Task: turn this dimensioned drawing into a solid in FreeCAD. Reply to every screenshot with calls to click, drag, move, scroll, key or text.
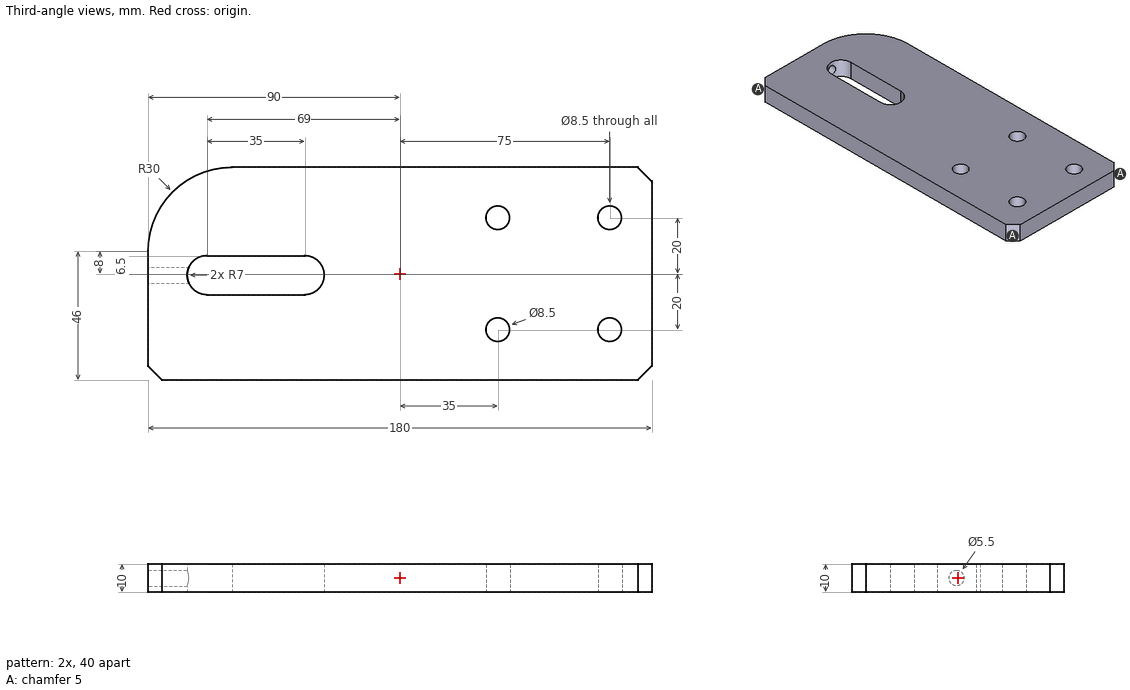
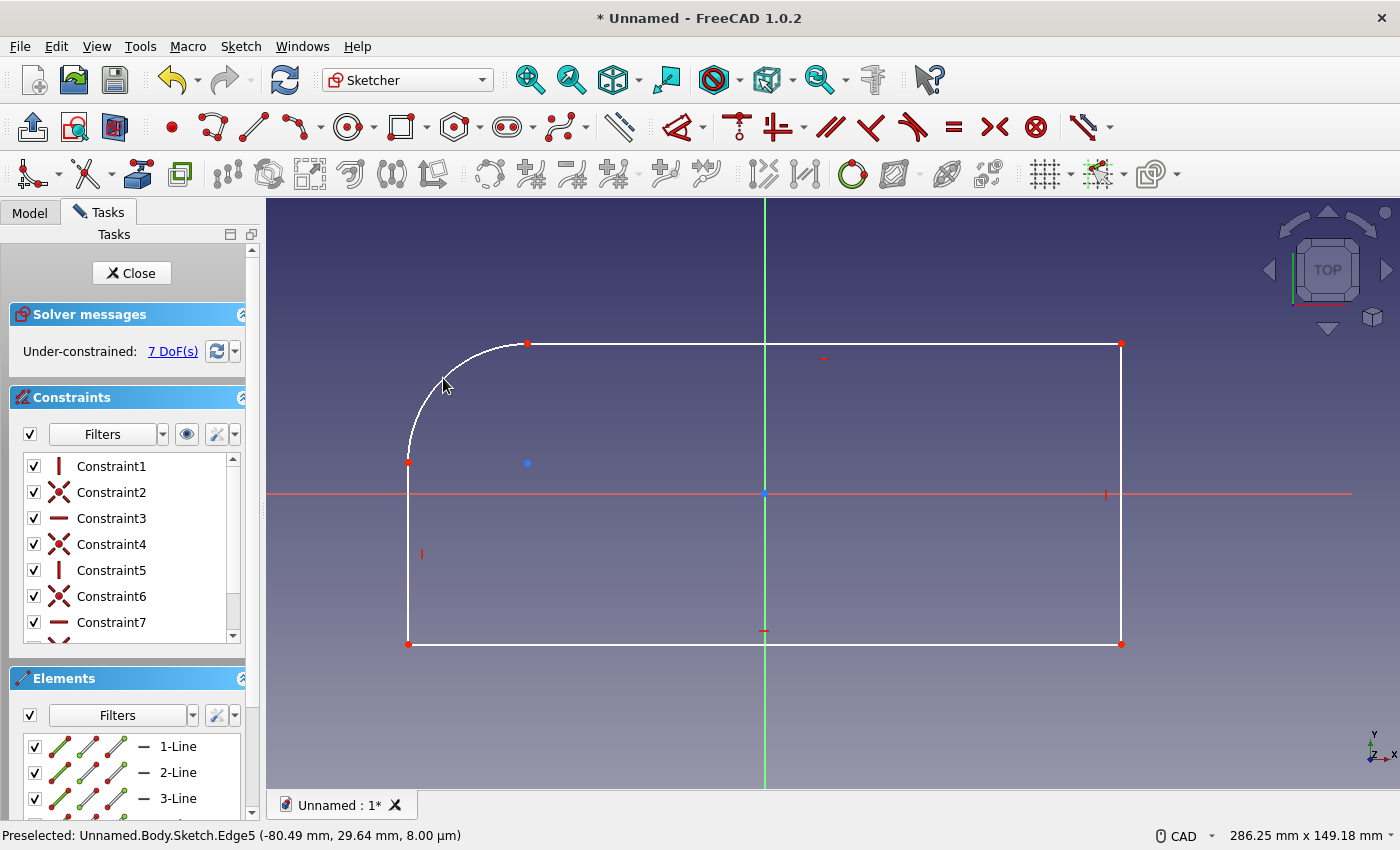
click(408, 518)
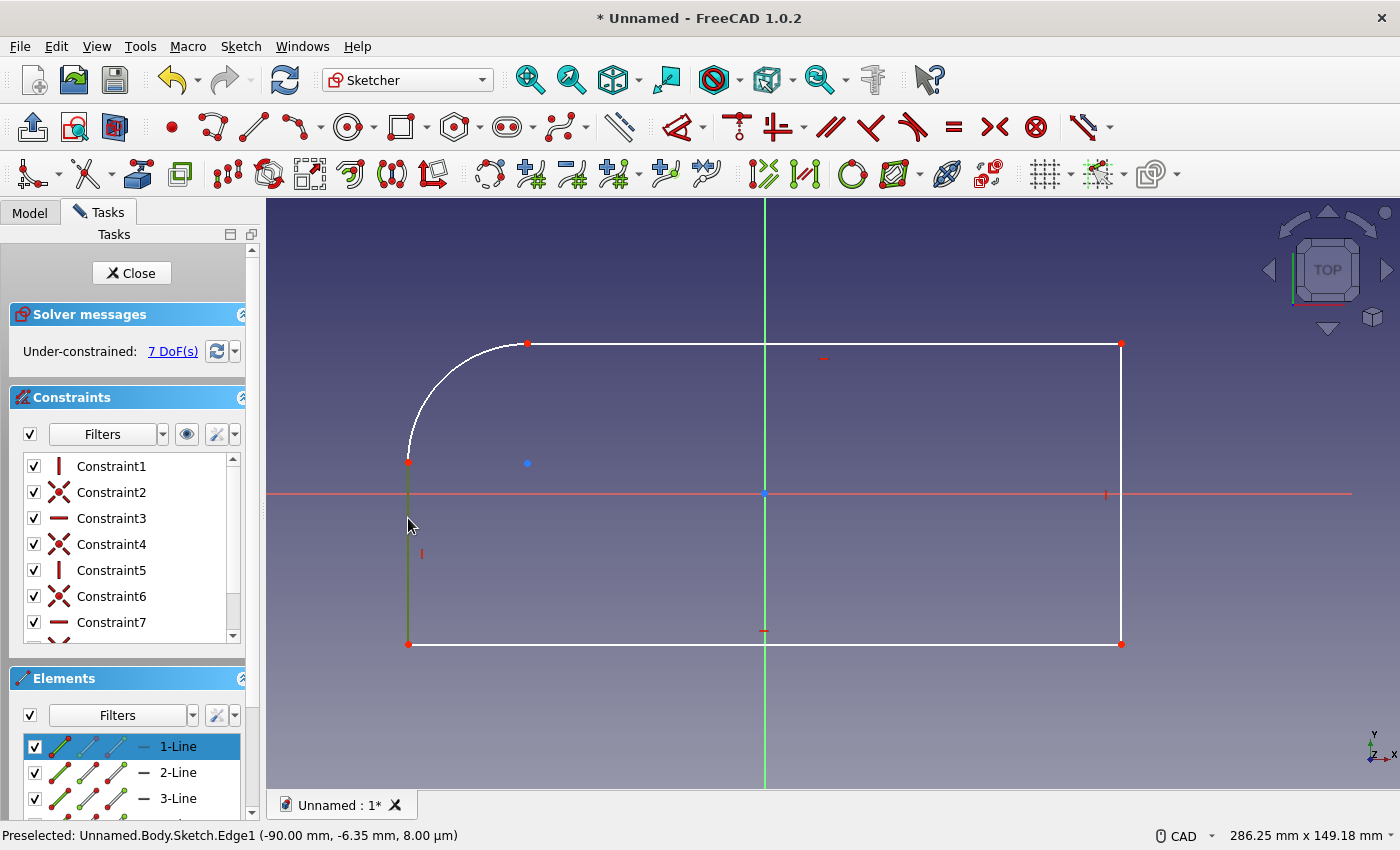
click(473, 357)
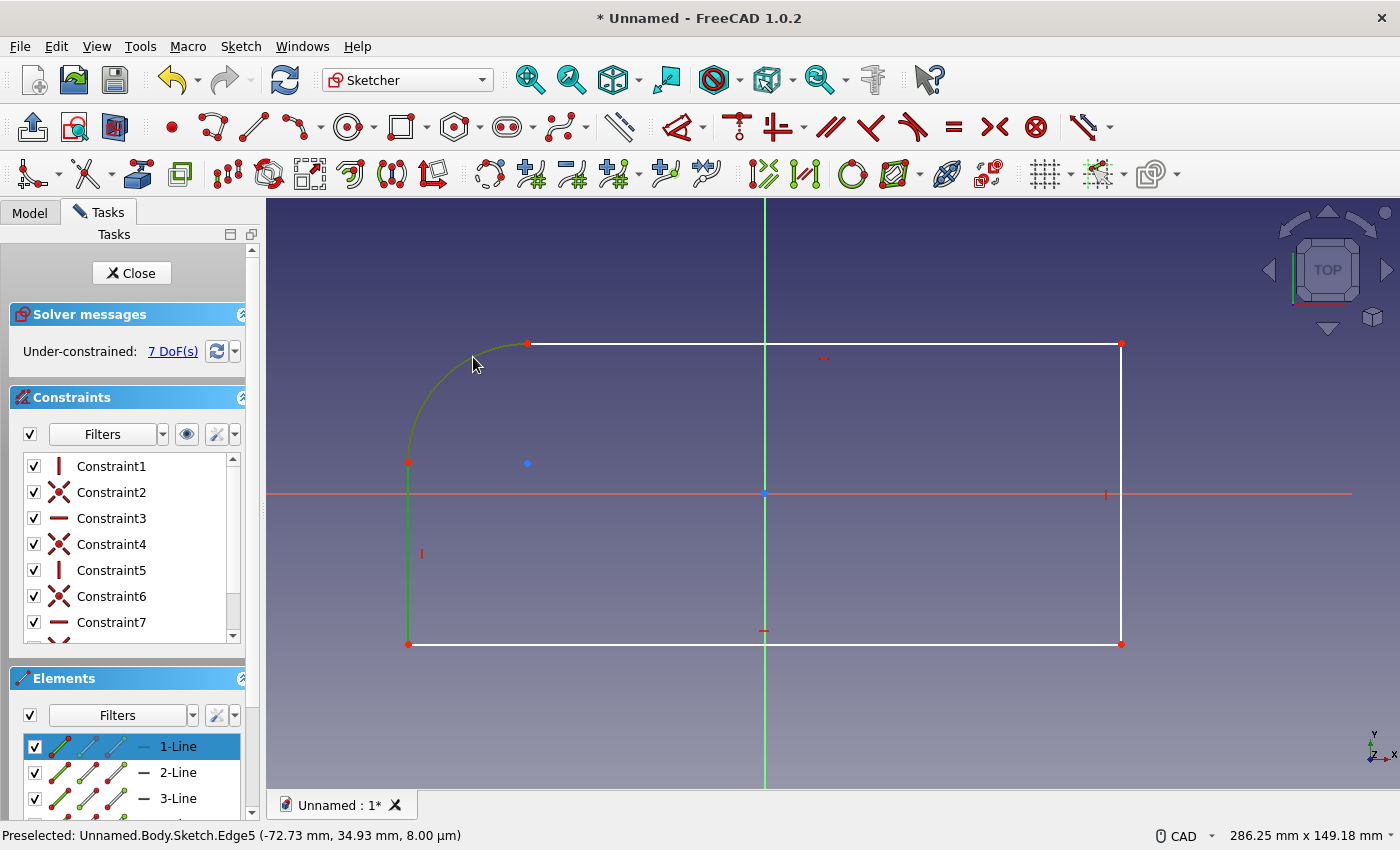
click(913, 128)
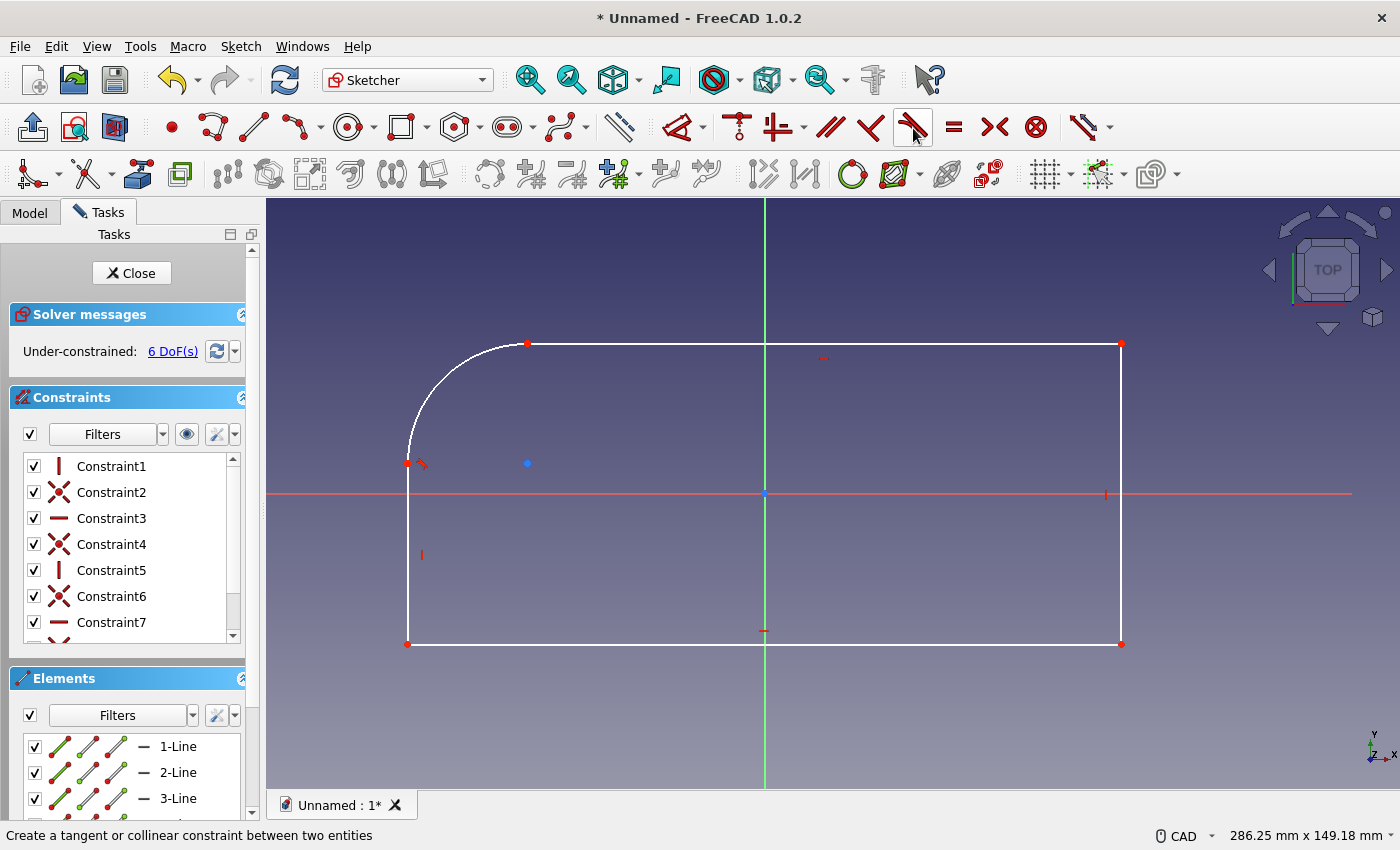
click(943, 344)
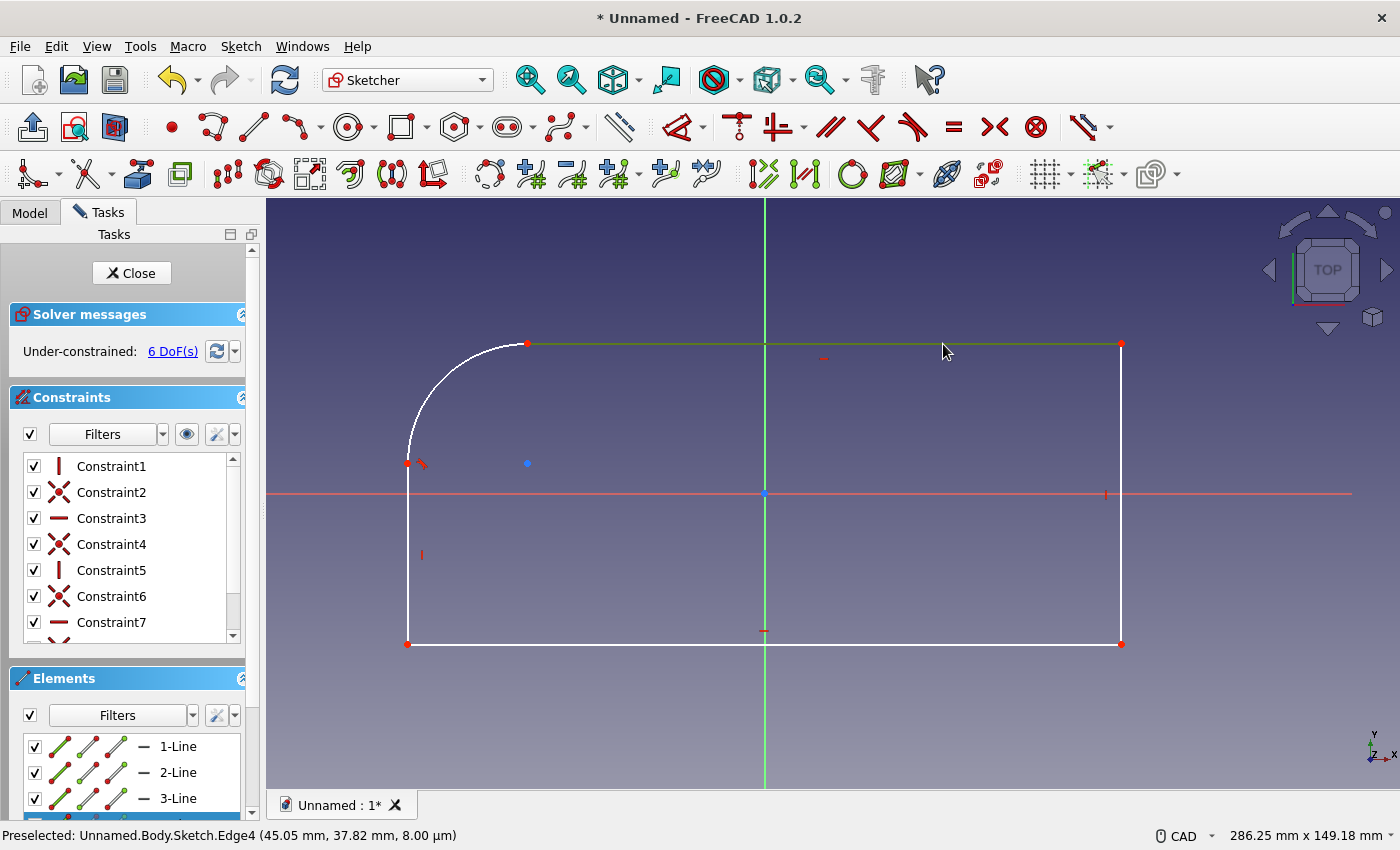
click(473, 357)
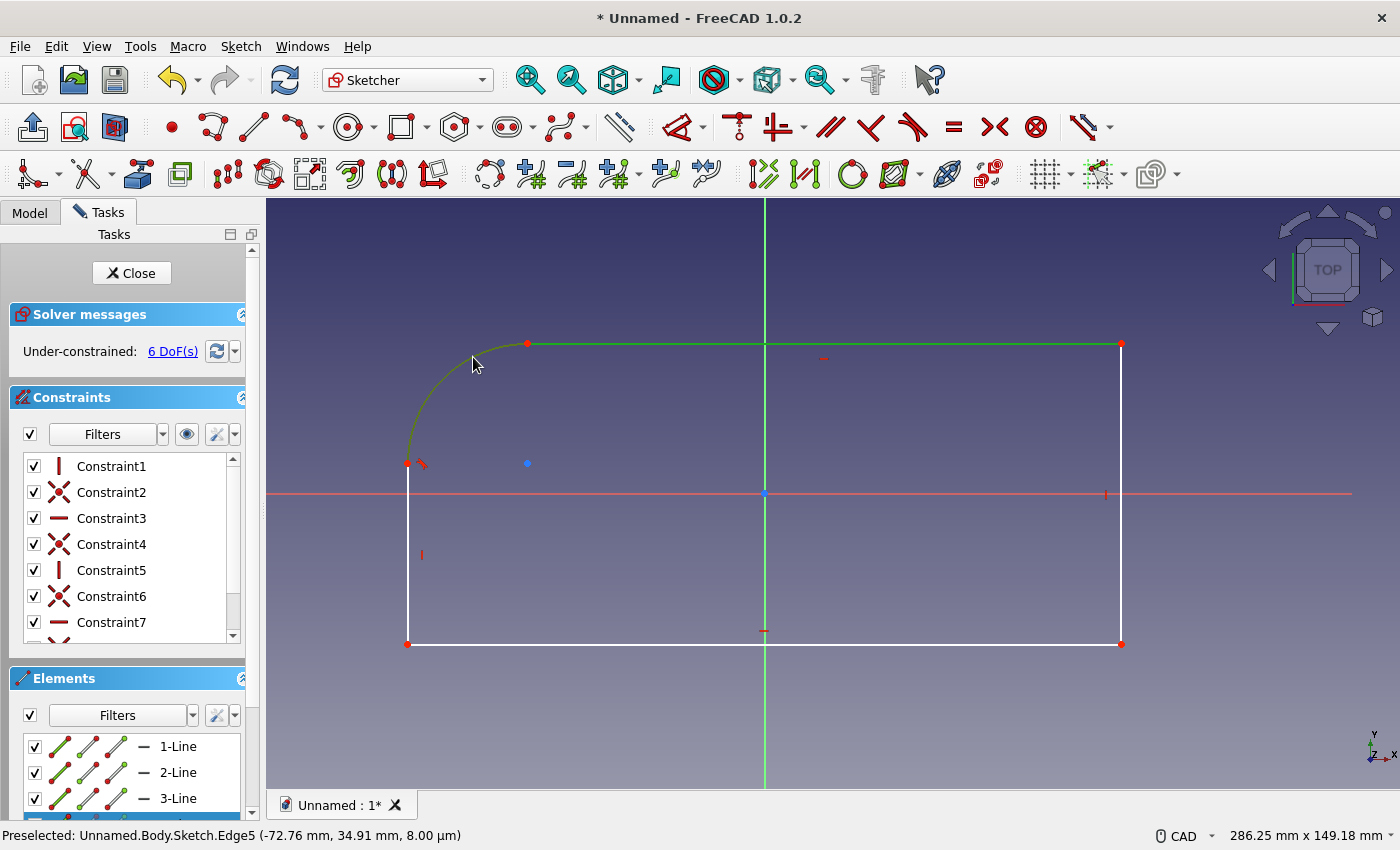
click(913, 128)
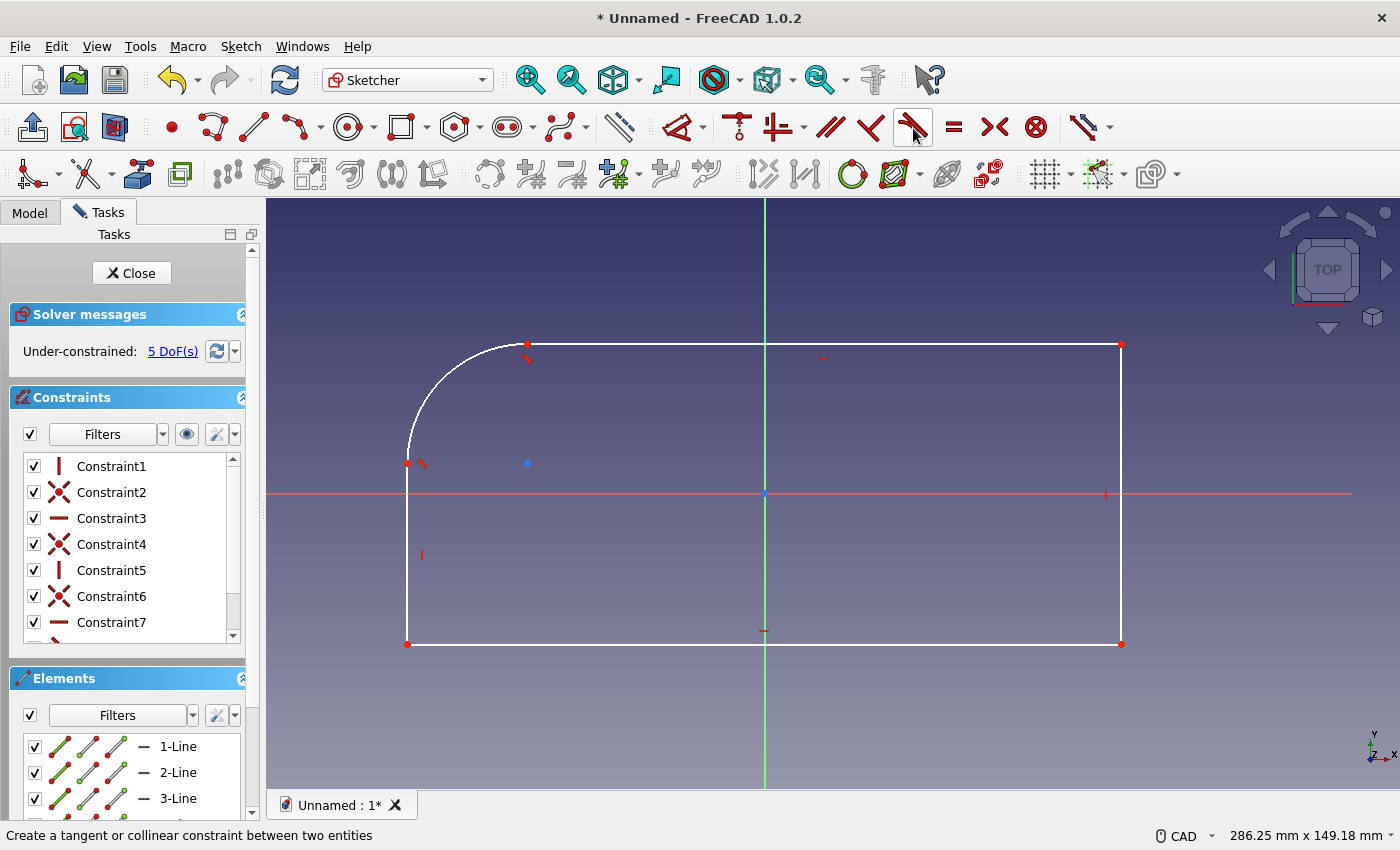
click(473, 357)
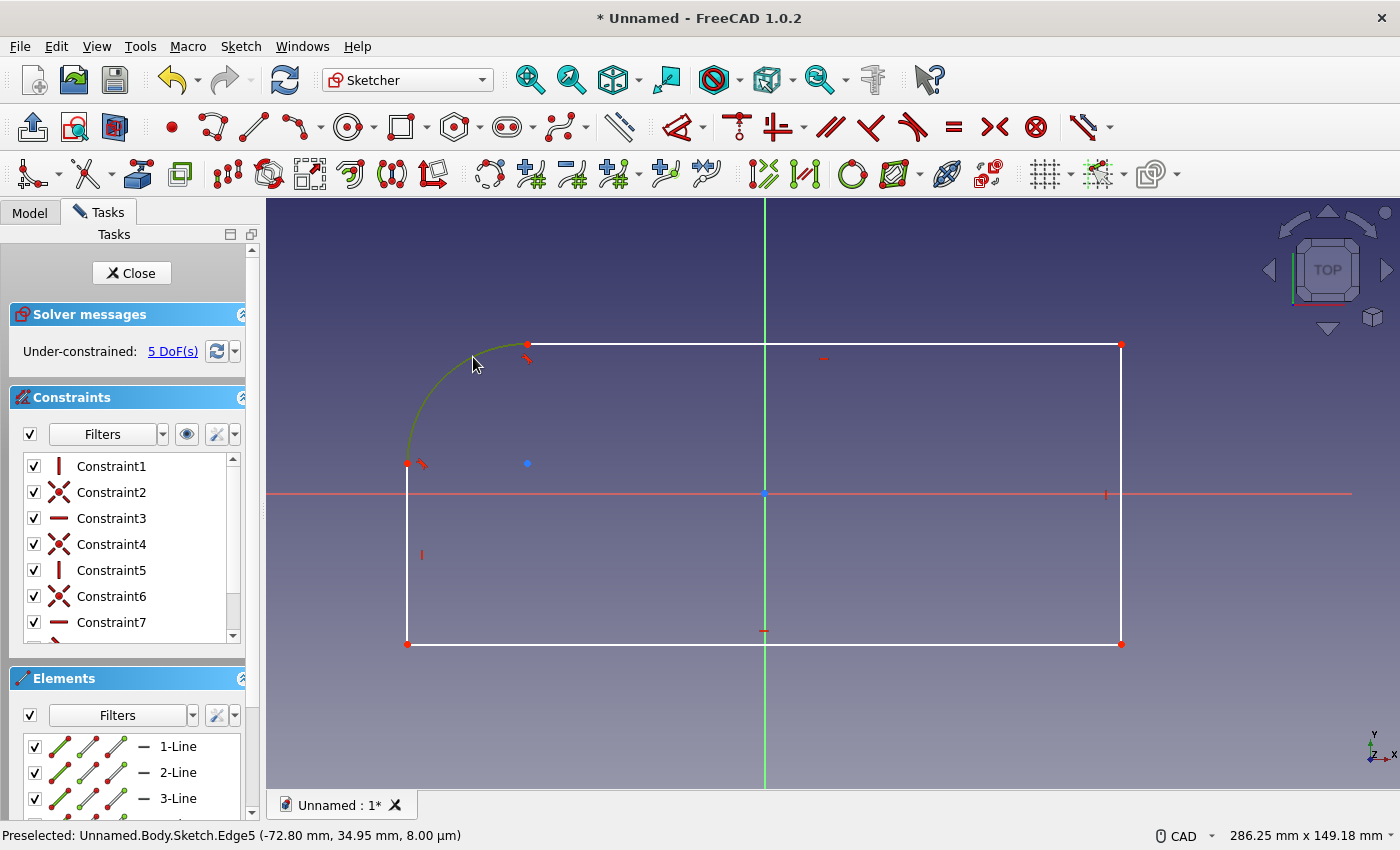
key(k)
key(r)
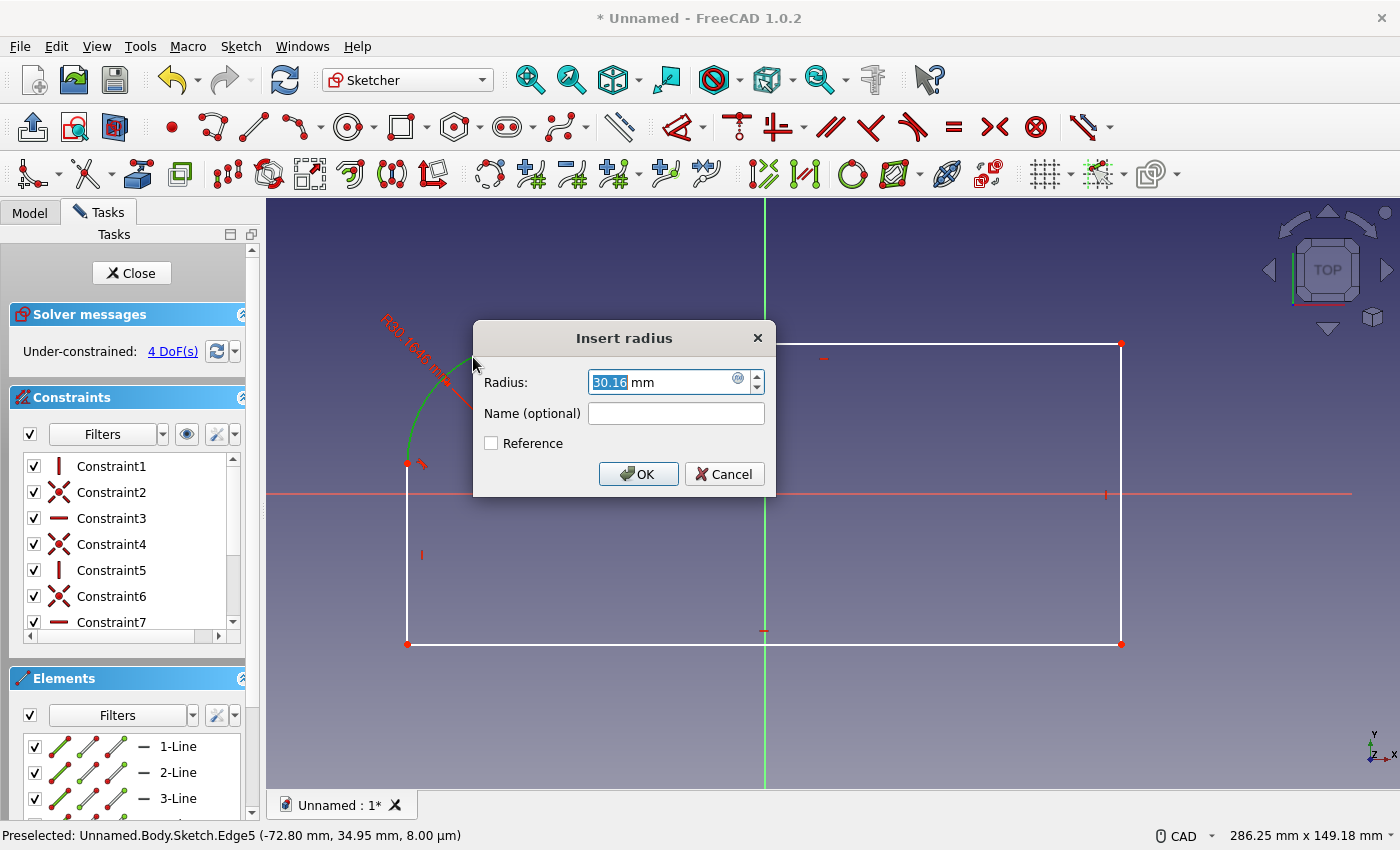
text(30)
key(Return)